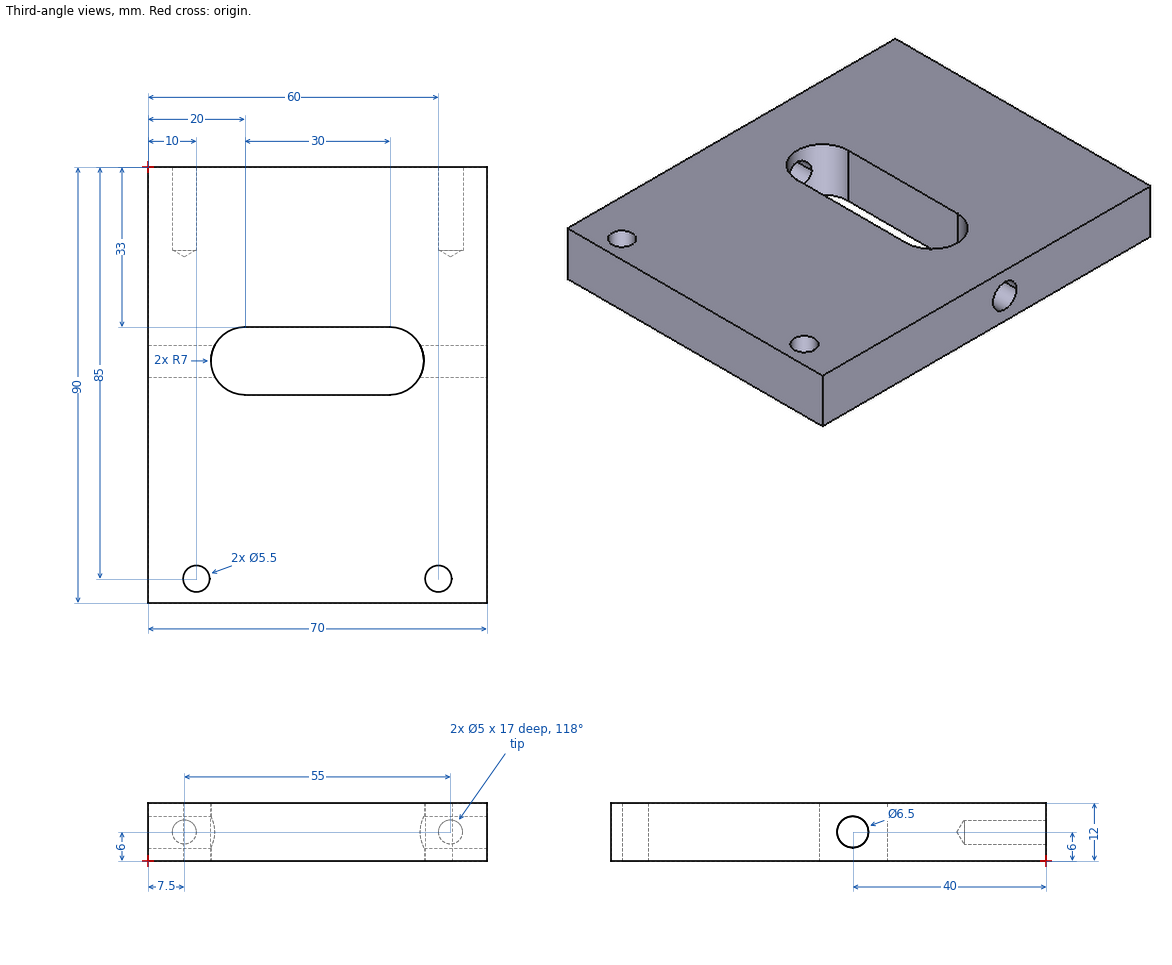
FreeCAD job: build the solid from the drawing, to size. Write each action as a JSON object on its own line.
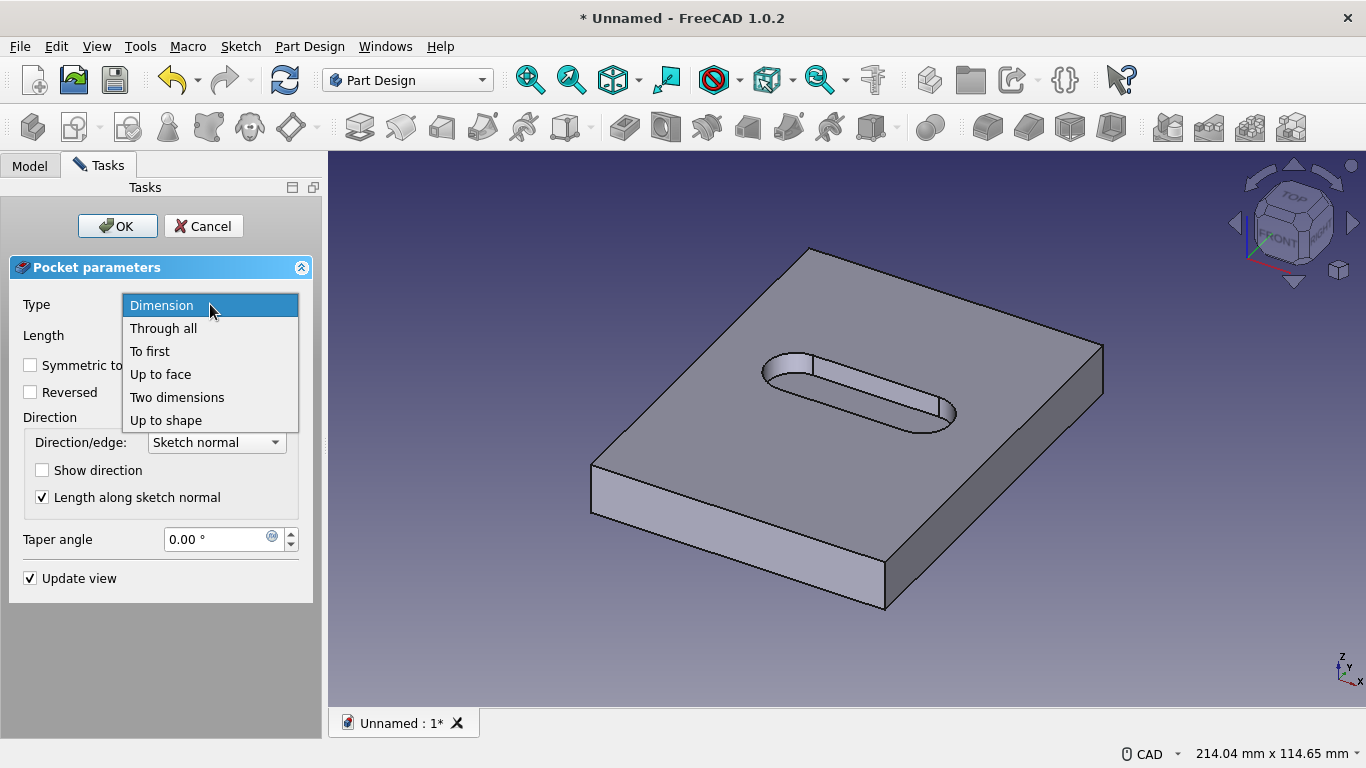
{"action": "left_click", "coordinate": [208, 328]}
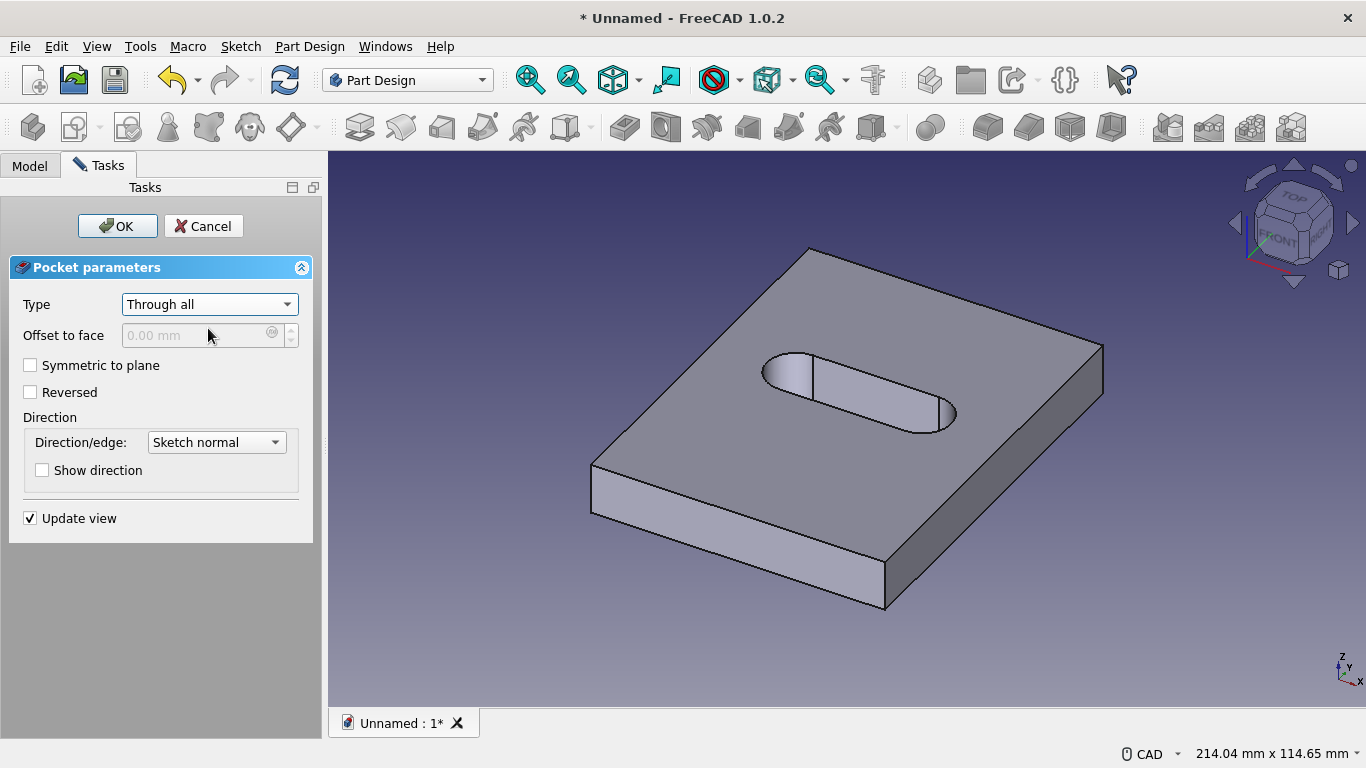
{"action": "left_click", "coordinate": [118, 226]}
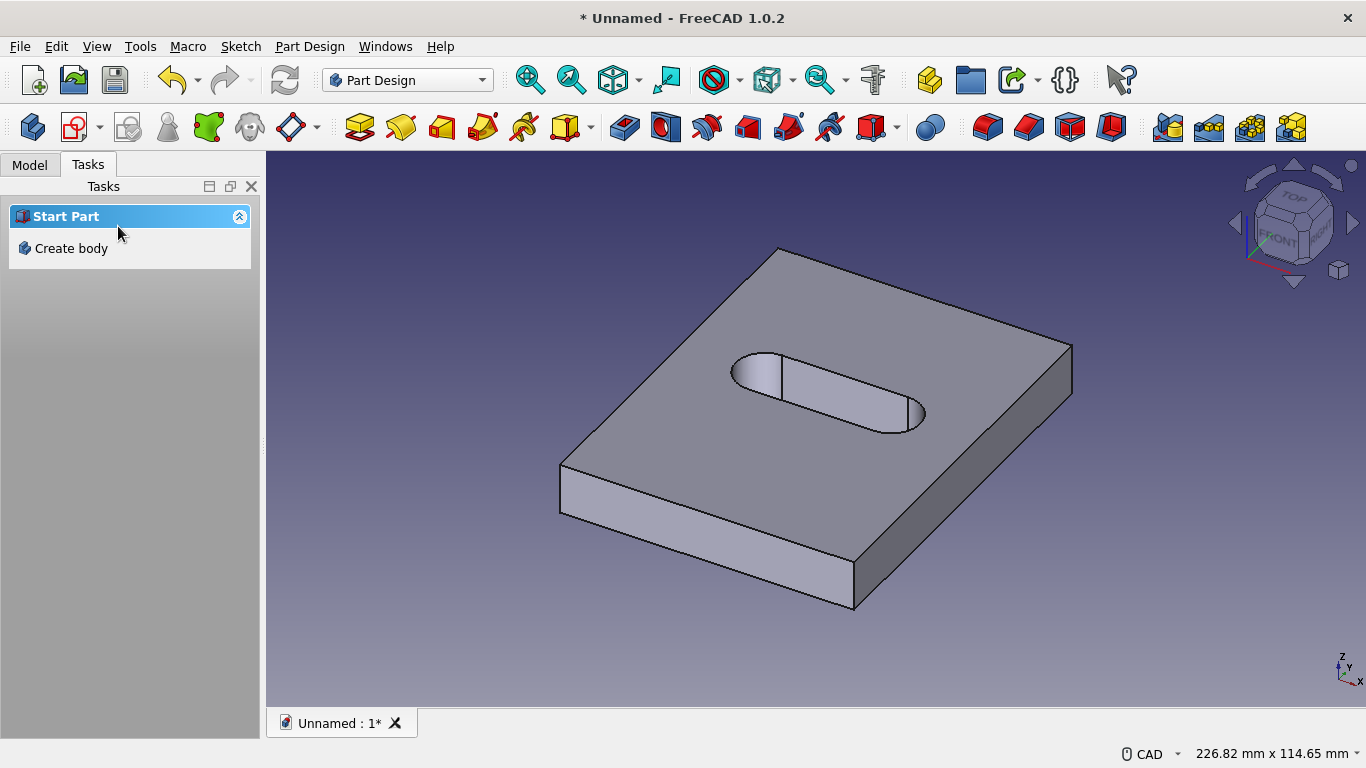
{"action": "left_click", "coordinate": [1057, 384]}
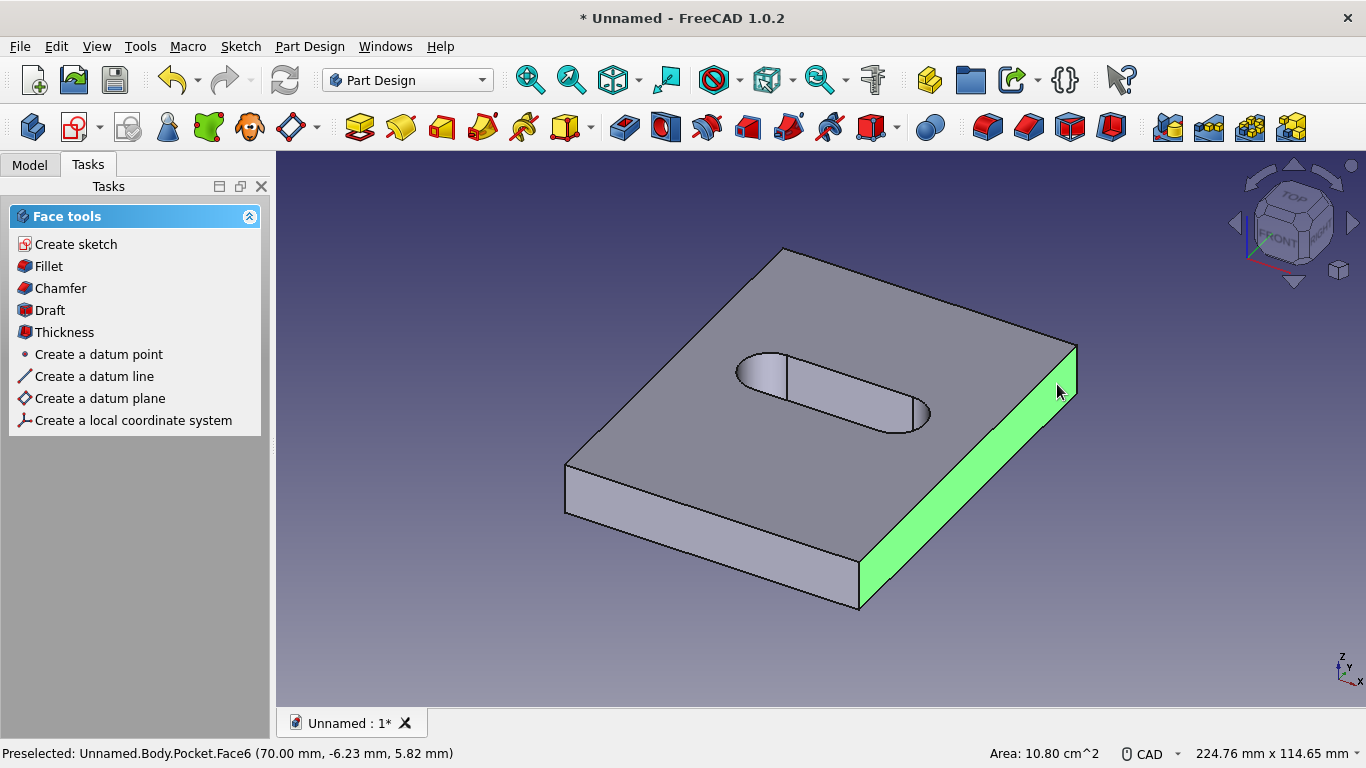
{"action": "left_click", "coordinate": [74, 128]}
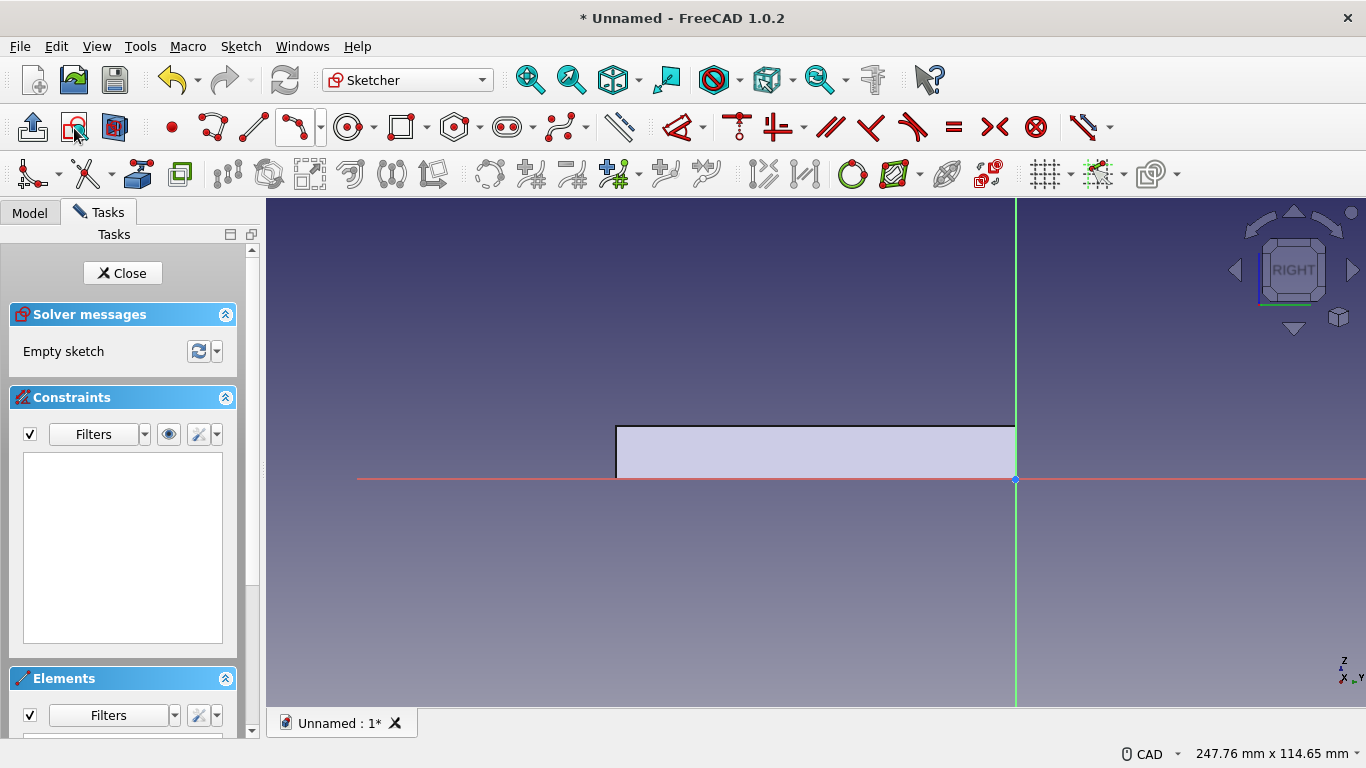
{"action": "scroll", "coordinate": [847, 452], "scroll_direction": "up", "scroll_amount": 12}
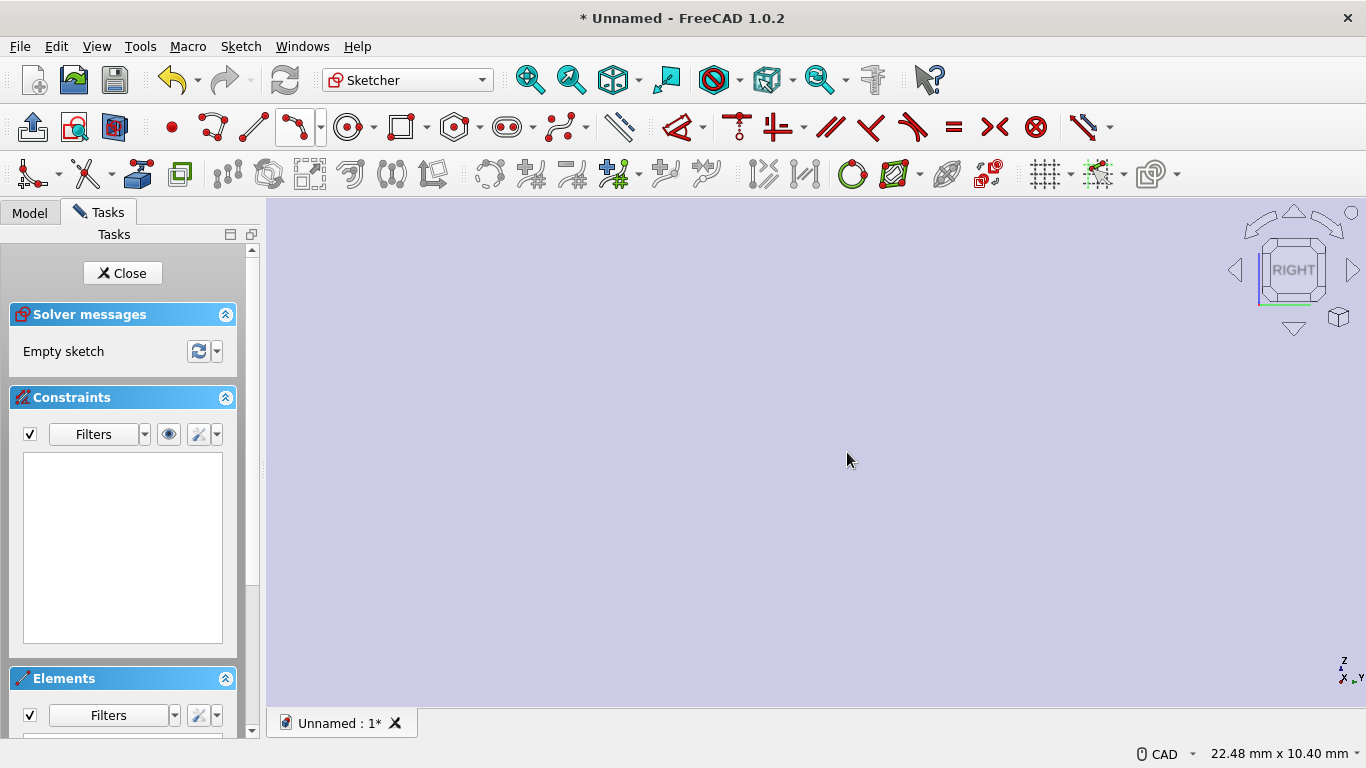
{"action": "left_click", "coordinate": [348, 128]}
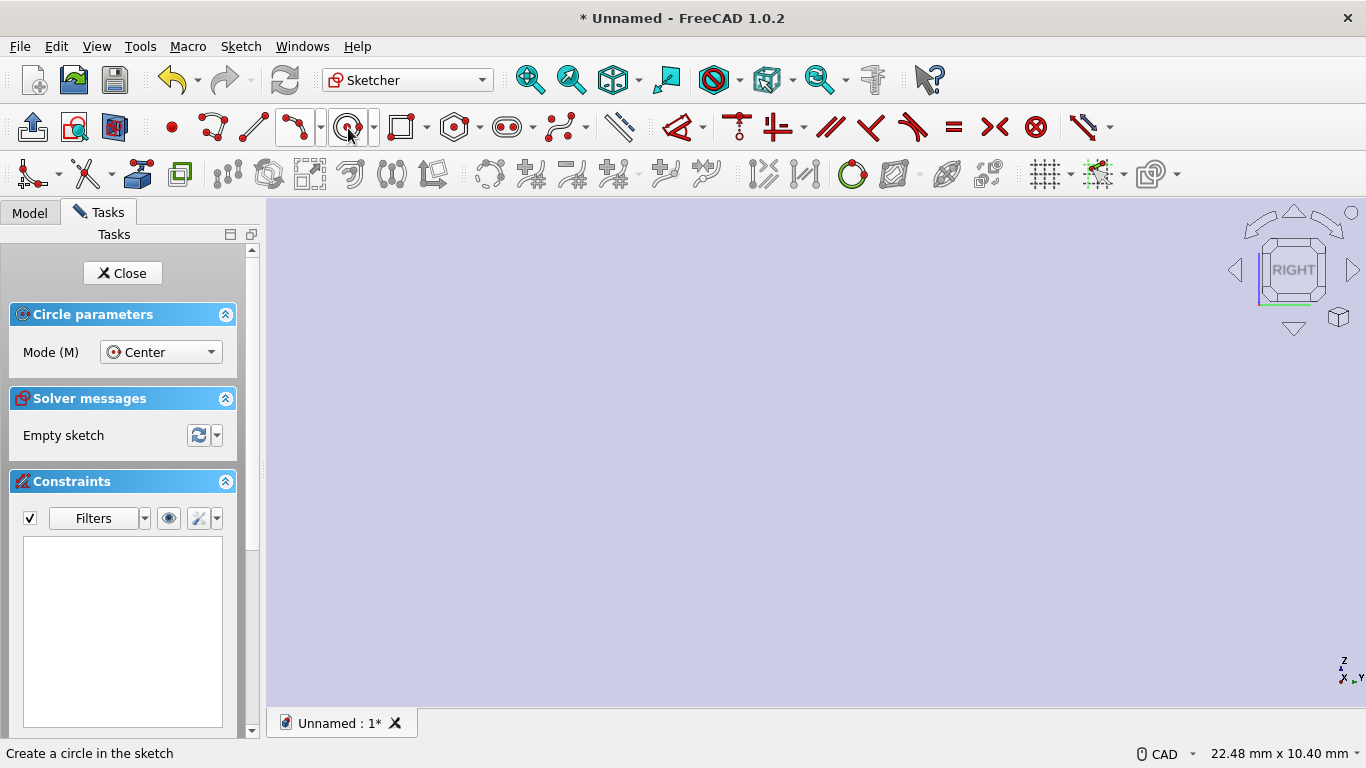
{"action": "left_click", "coordinate": [745, 452]}
{"action": "left_click", "coordinate": [857, 340]}
{"action": "key", "text": "Escape"}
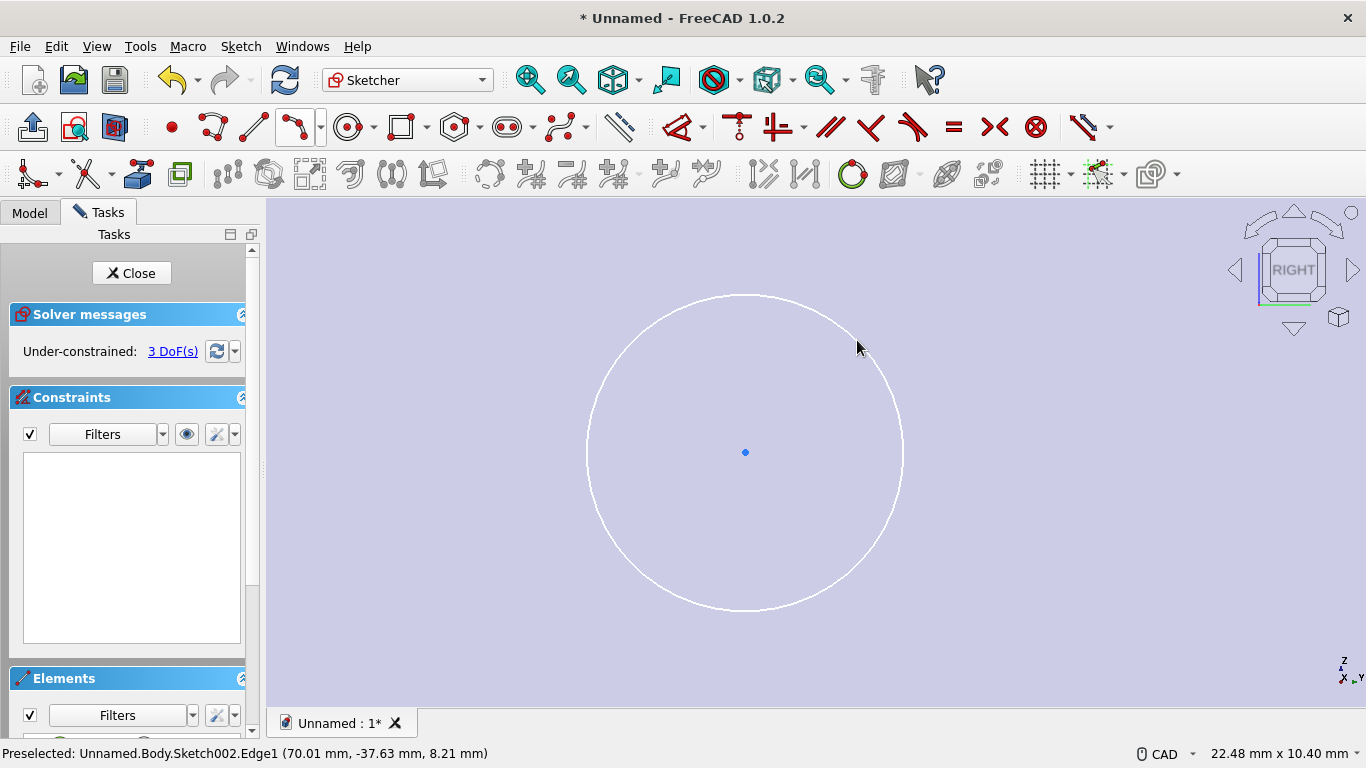
{"action": "left_click", "coordinate": [676, 128]}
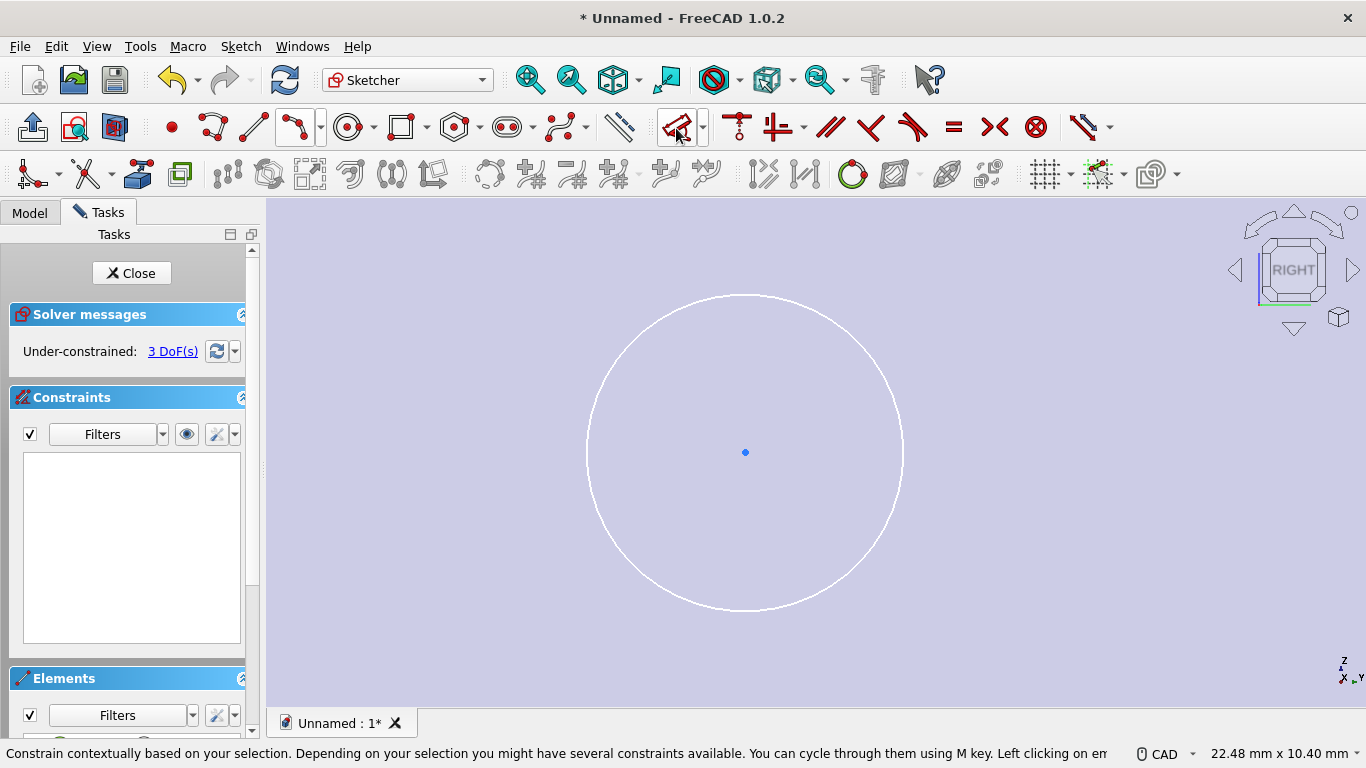
{"action": "left_click", "coordinate": [857, 341]}
{"action": "left_click", "coordinate": [880, 318]}